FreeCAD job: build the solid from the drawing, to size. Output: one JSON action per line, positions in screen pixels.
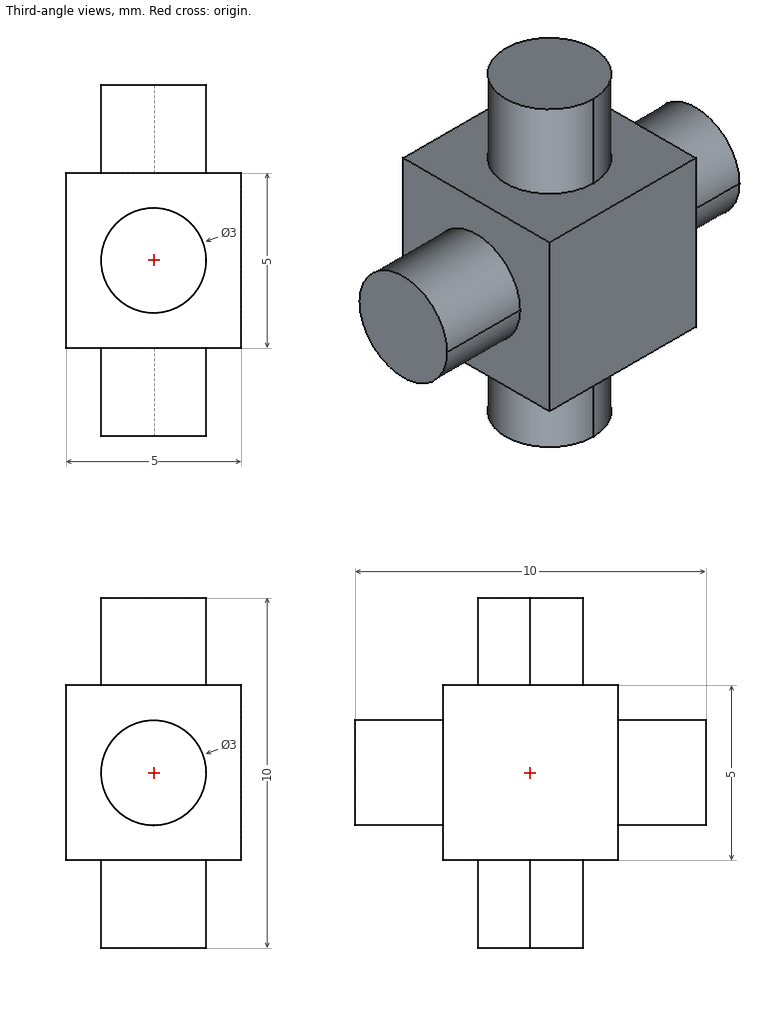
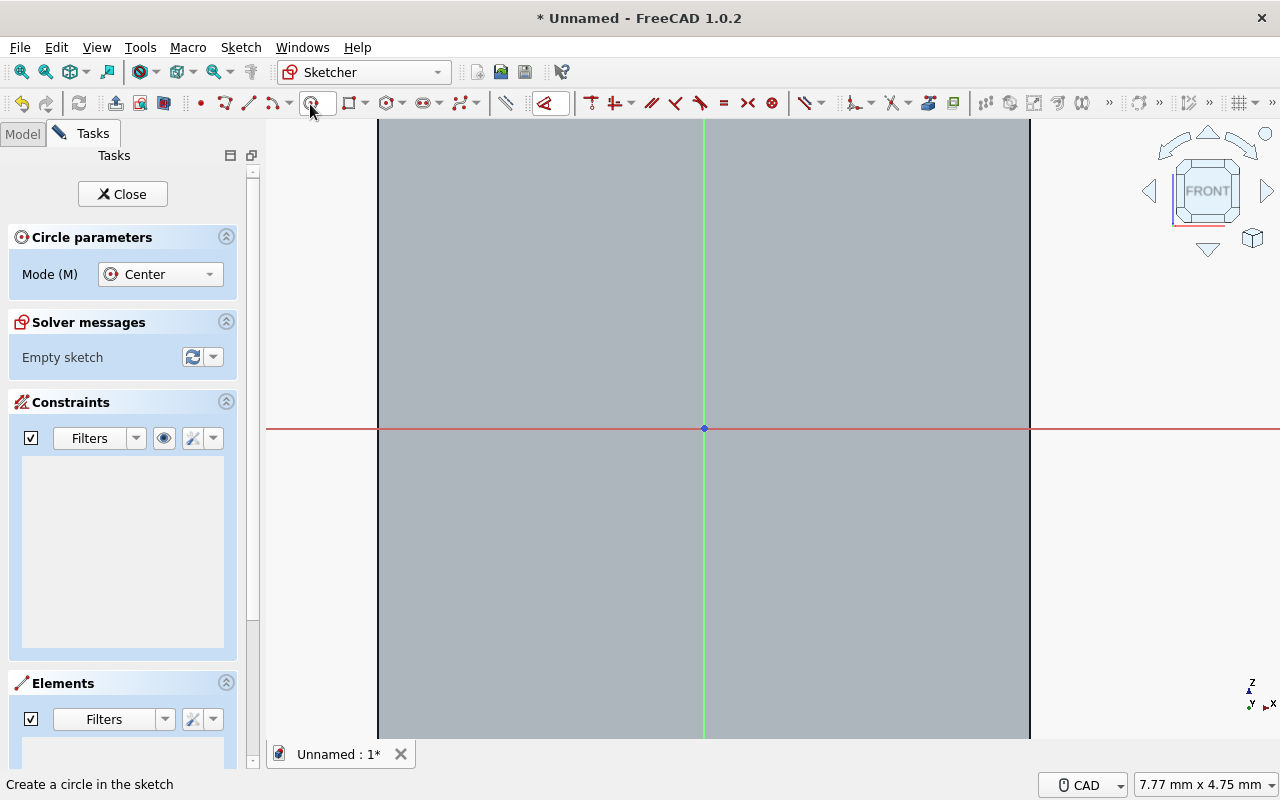
{"action": "left_click", "coordinate": [704, 429]}
{"action": "mouse_move", "coordinate": [843, 290]}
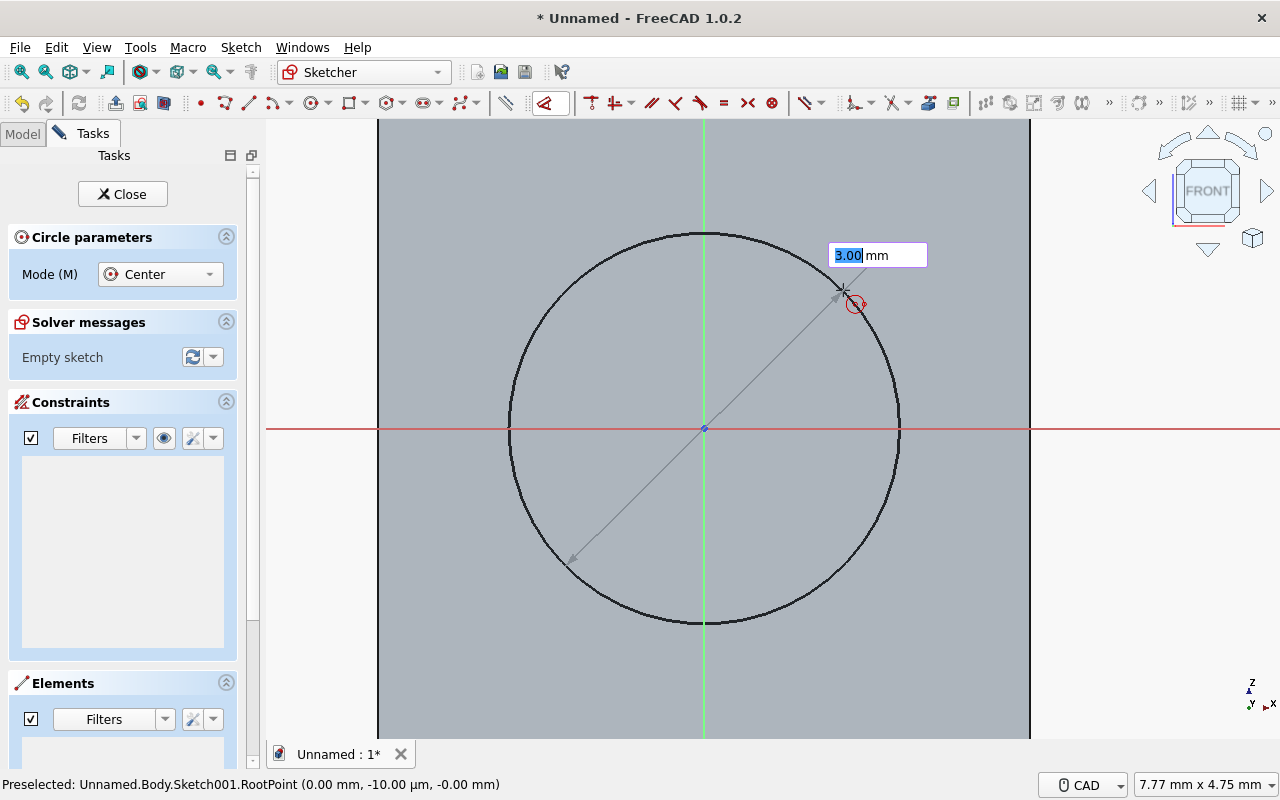
{"action": "type", "text": "3"}
{"action": "key", "text": "Return"}
{"action": "key", "text": "Escape"}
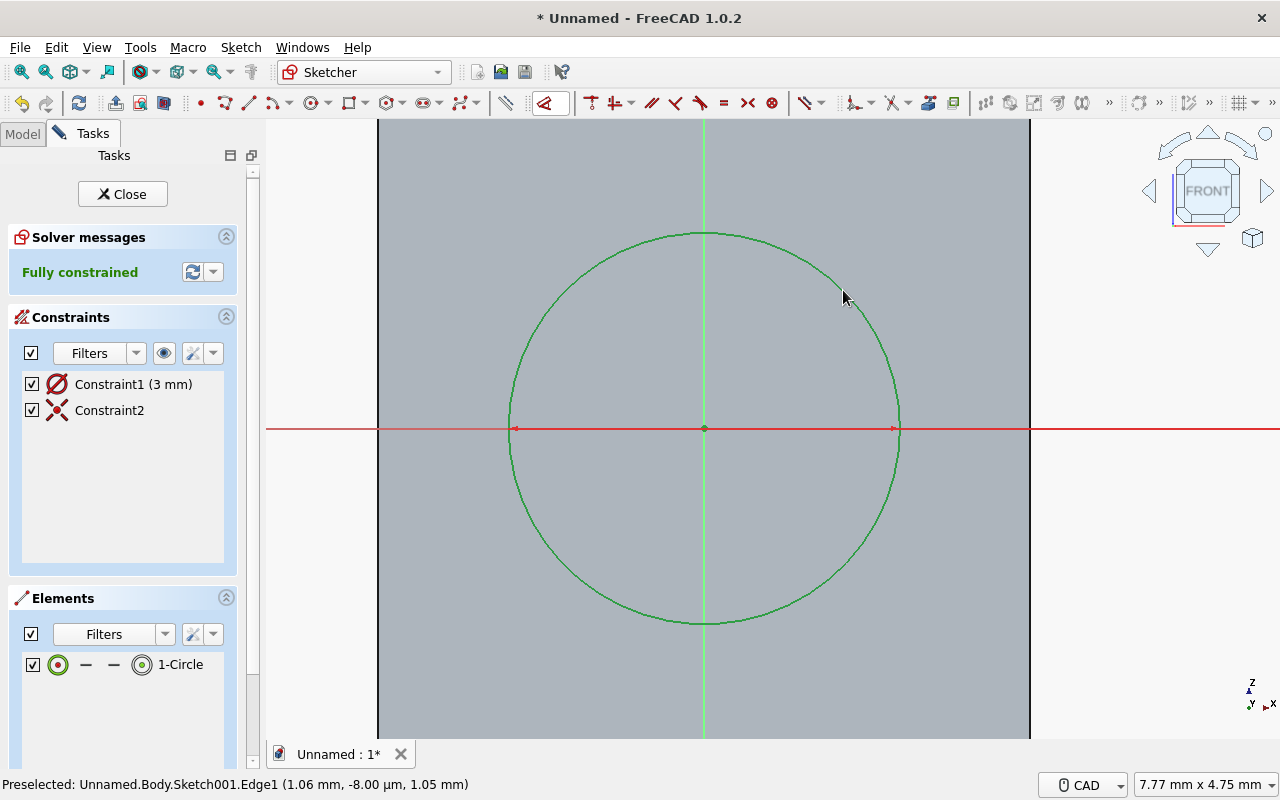
{"action": "left_click", "coordinate": [123, 194]}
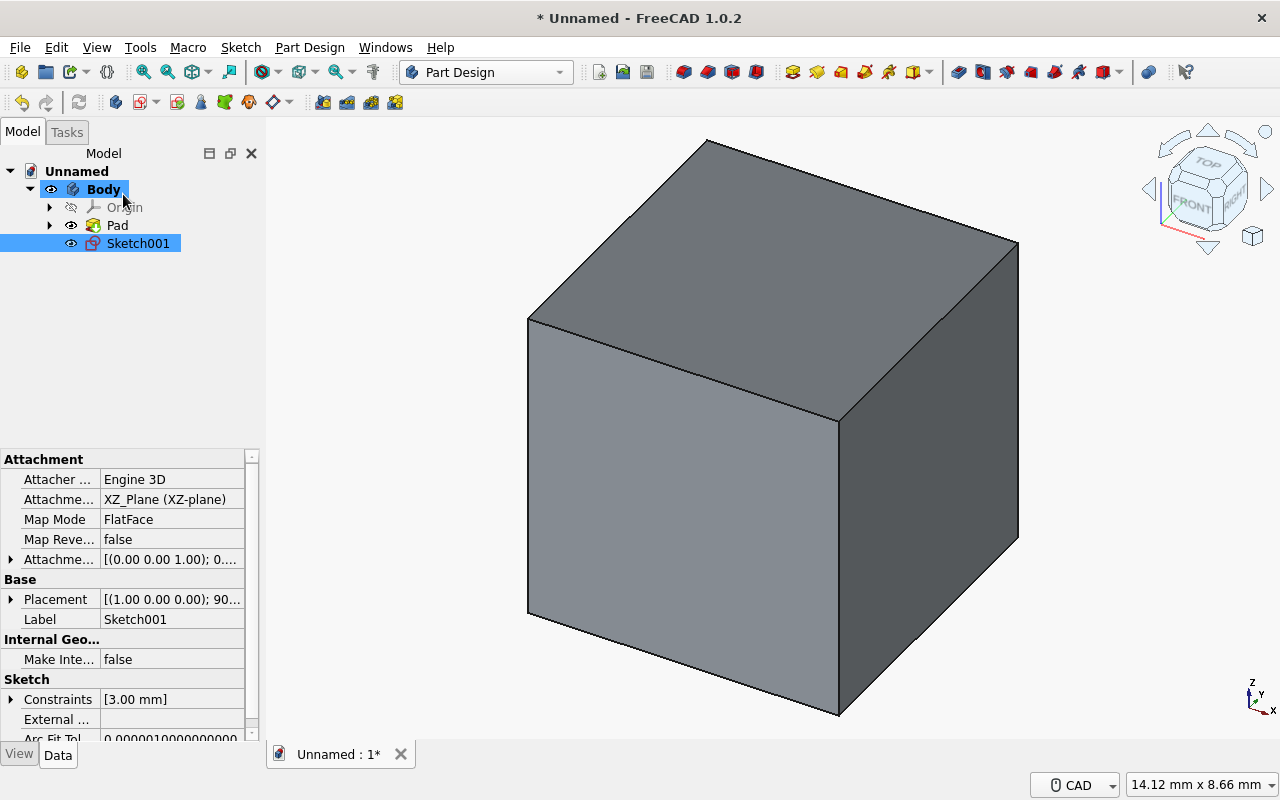
{"action": "left_click", "coordinate": [794, 72]}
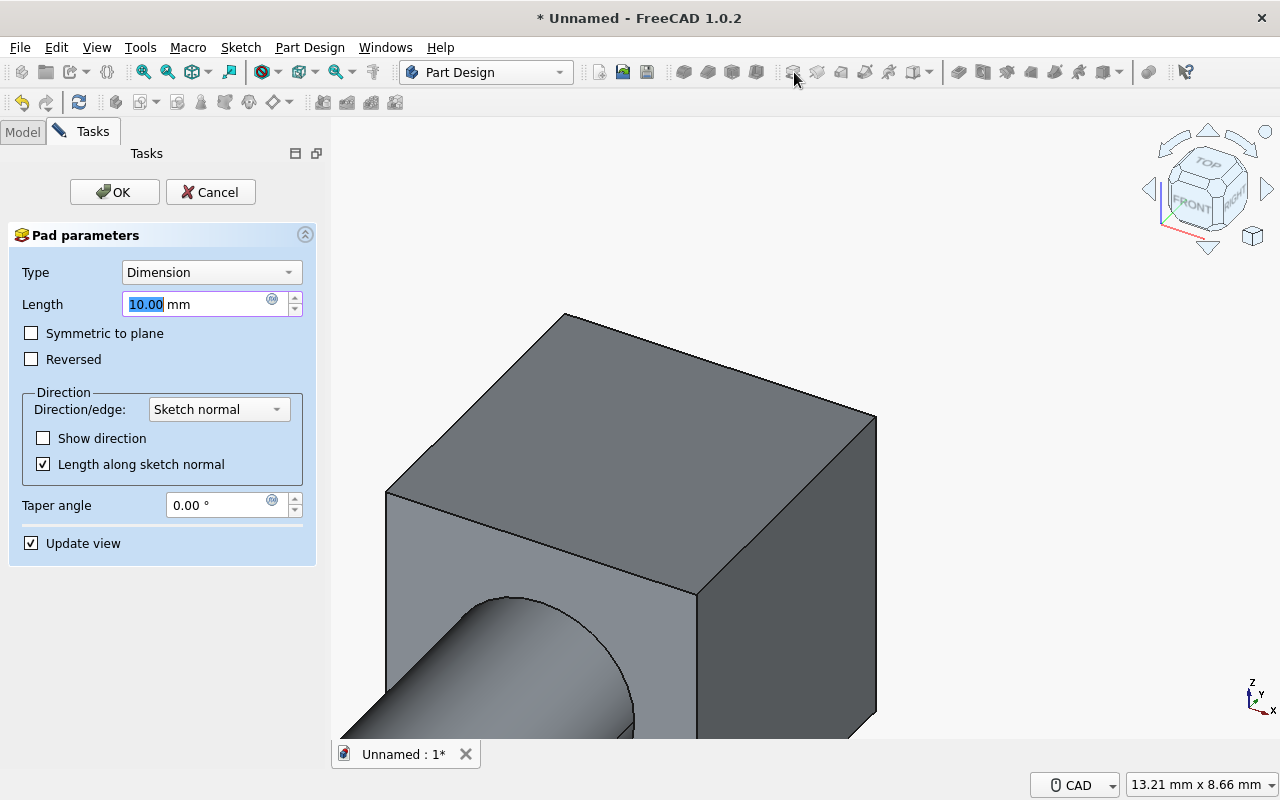
{"action": "type", "text": "10"}
{"action": "key", "text": "Tab"}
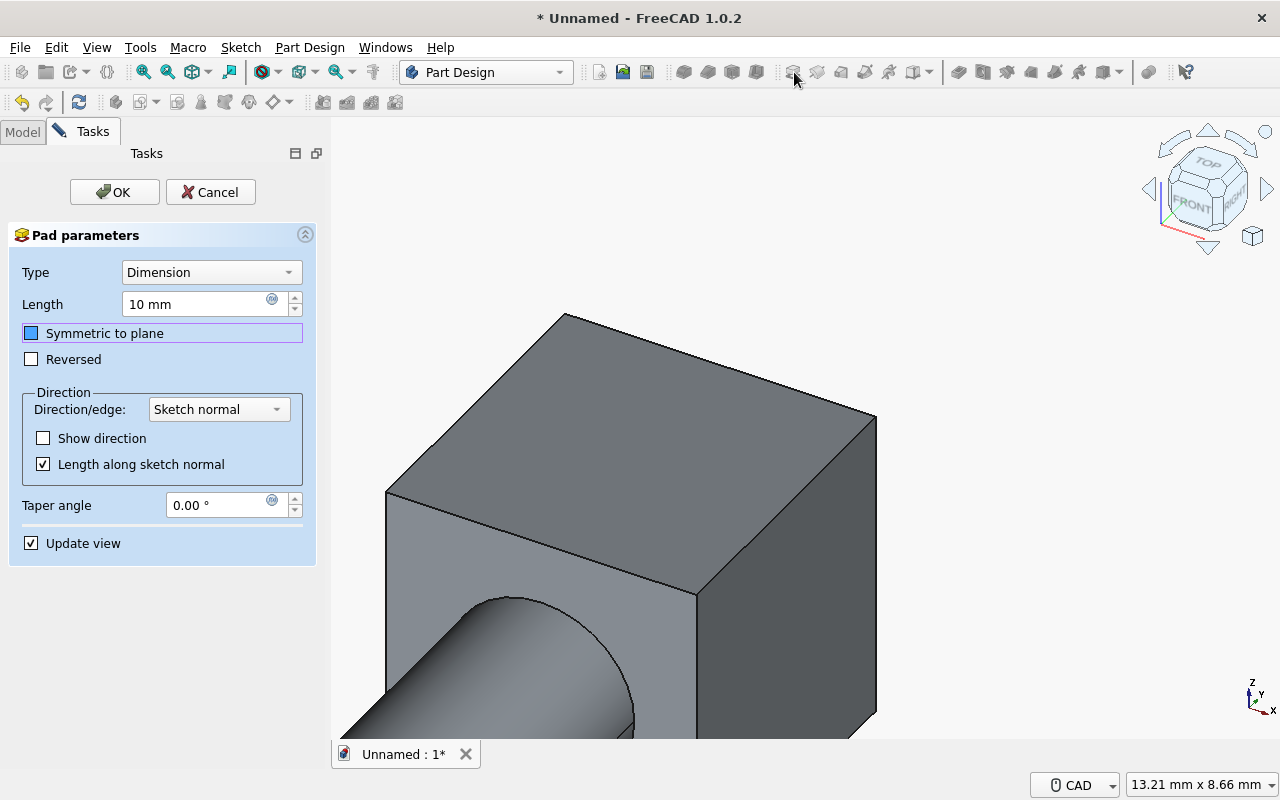
{"action": "left_click", "coordinate": [30, 333]}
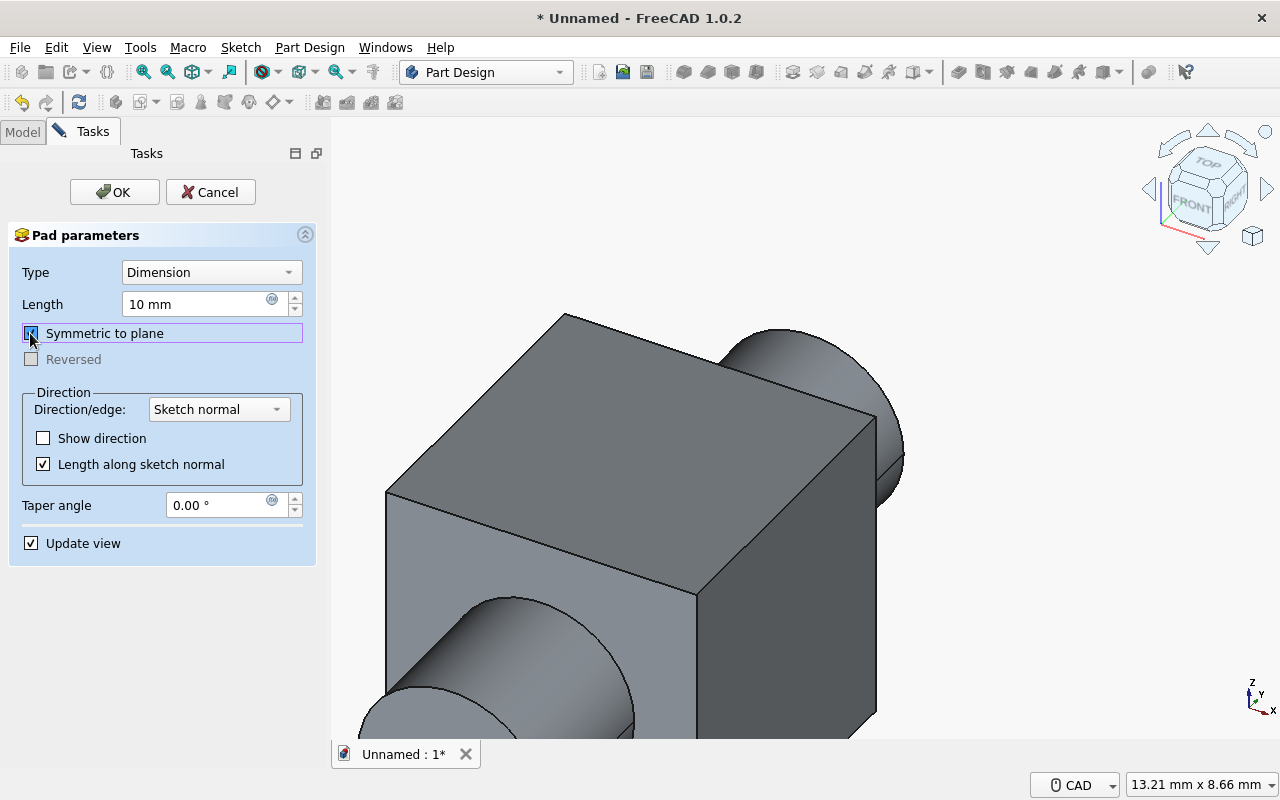
{"action": "left_click", "coordinate": [115, 192]}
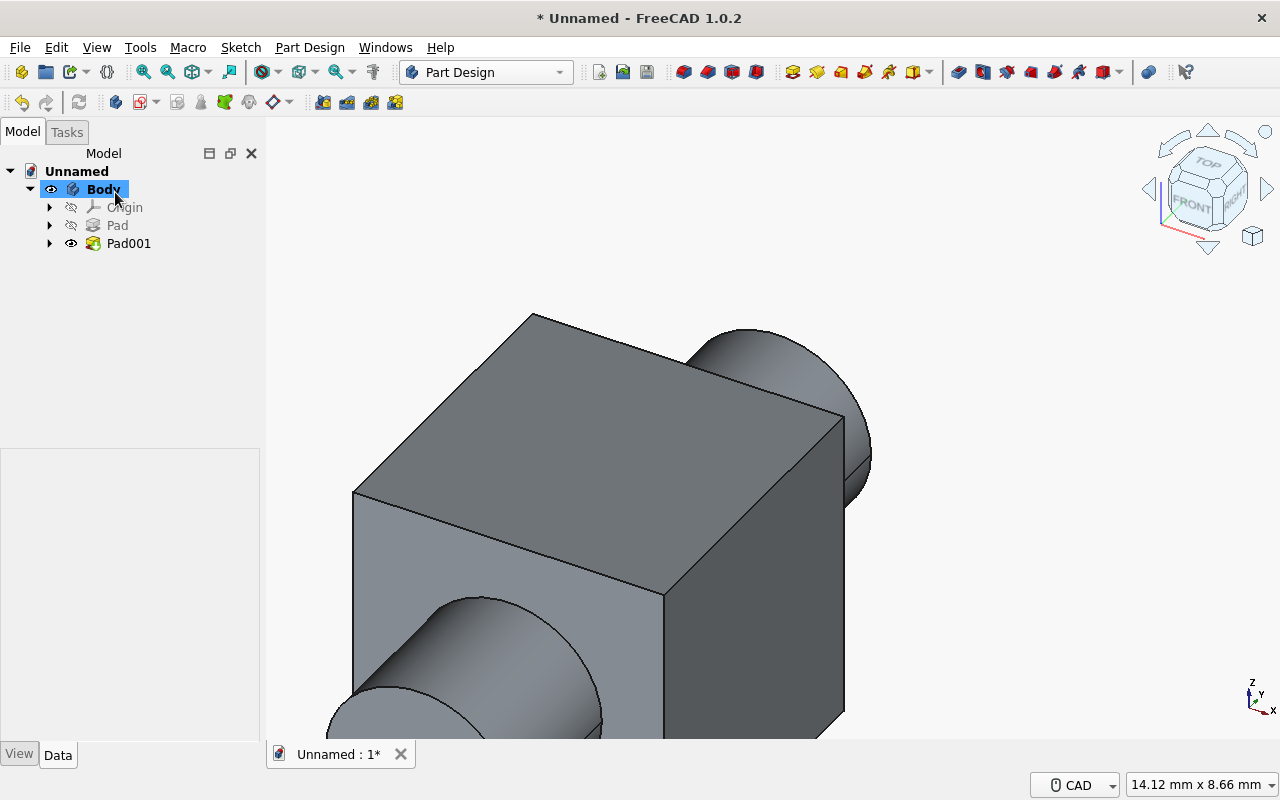
{"action": "left_click", "coordinate": [144, 72]}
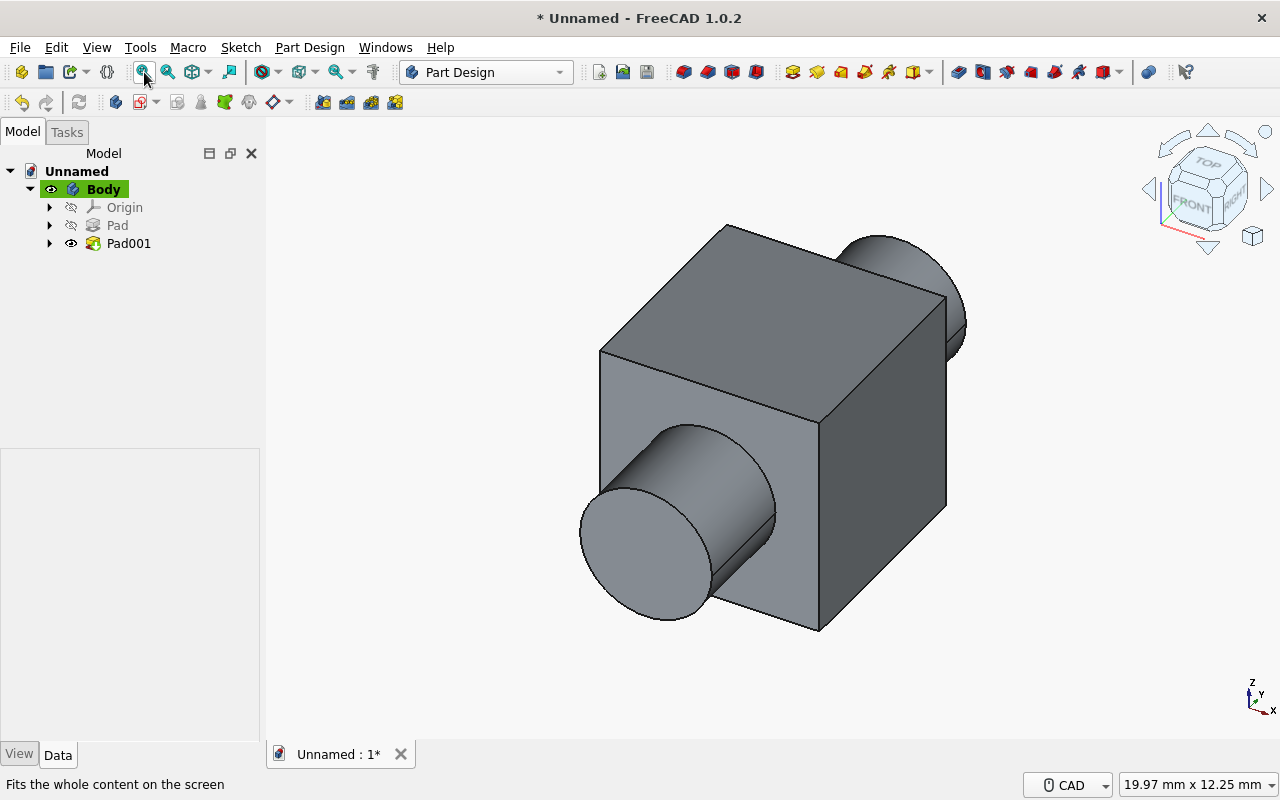
{"action": "left_click", "coordinate": [140, 102]}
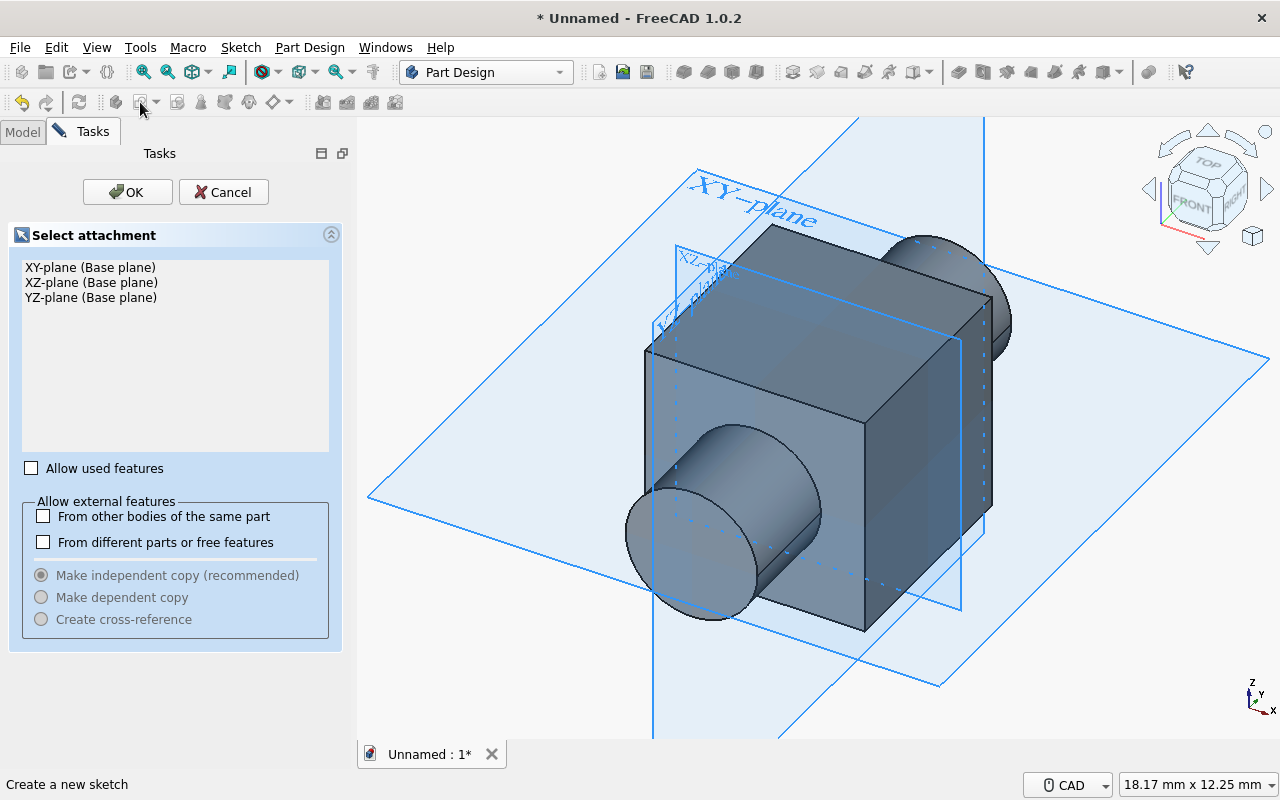
{"action": "left_click", "coordinate": [82, 268]}